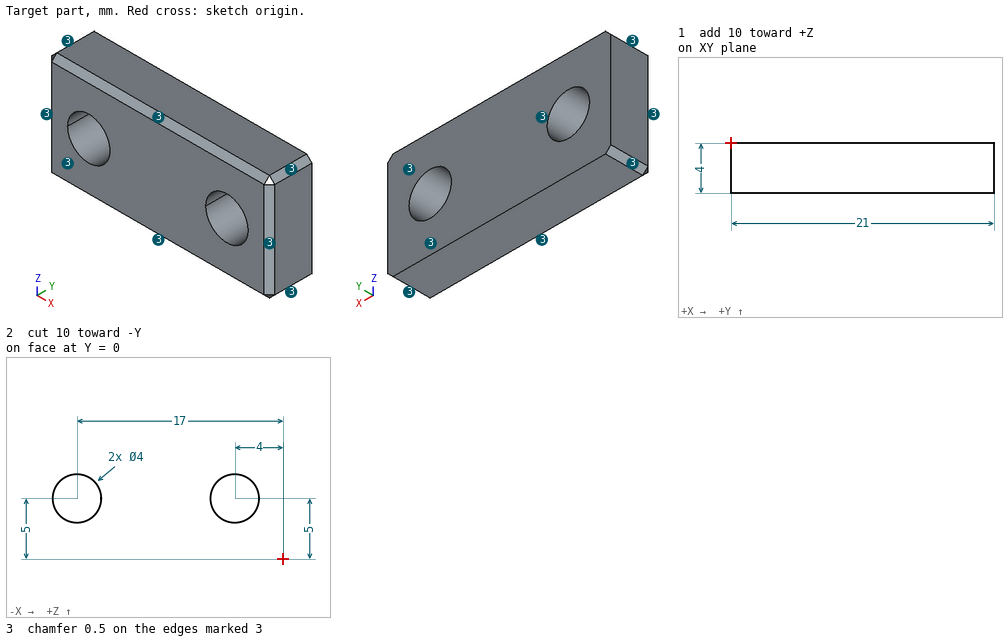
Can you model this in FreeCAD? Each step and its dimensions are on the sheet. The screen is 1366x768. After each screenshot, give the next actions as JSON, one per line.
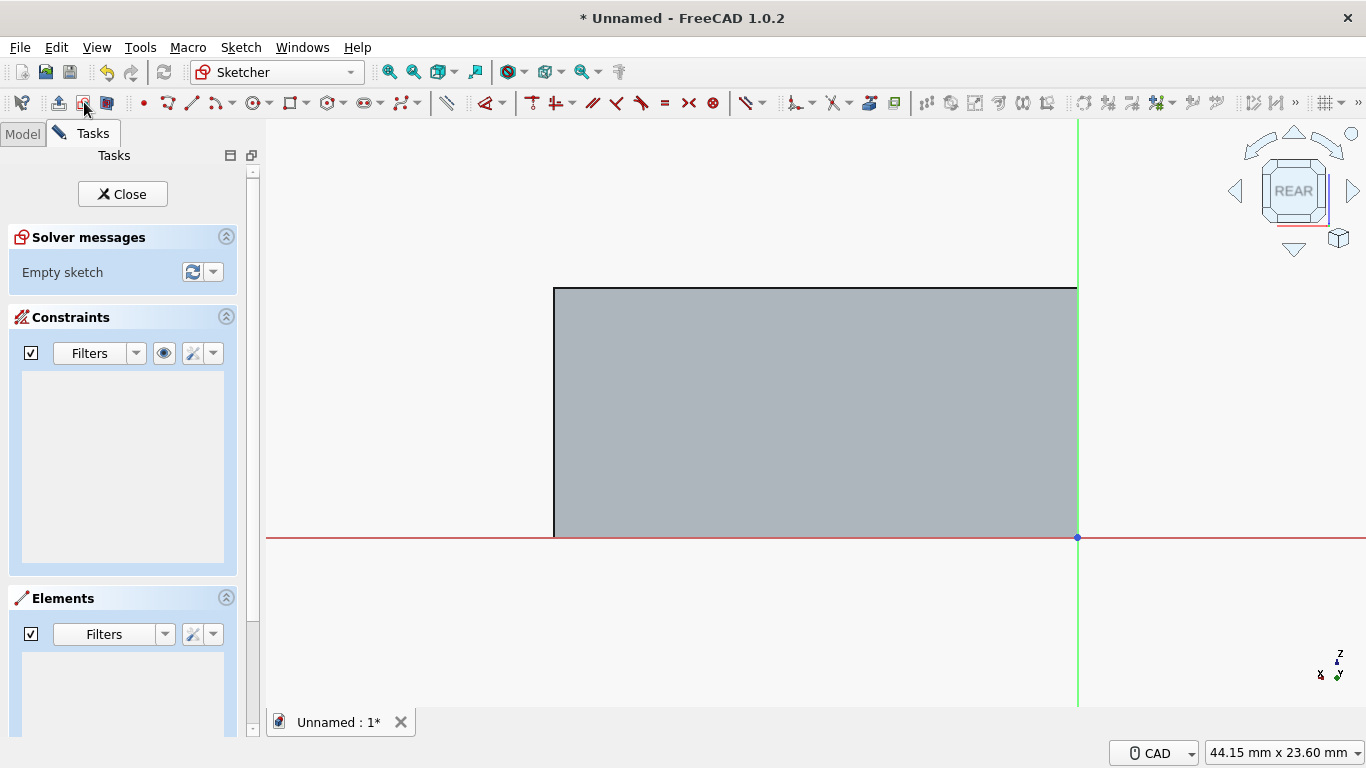
{"action": "scroll", "coordinate": [1031, 526], "scroll_direction": "up", "scroll_amount": 2}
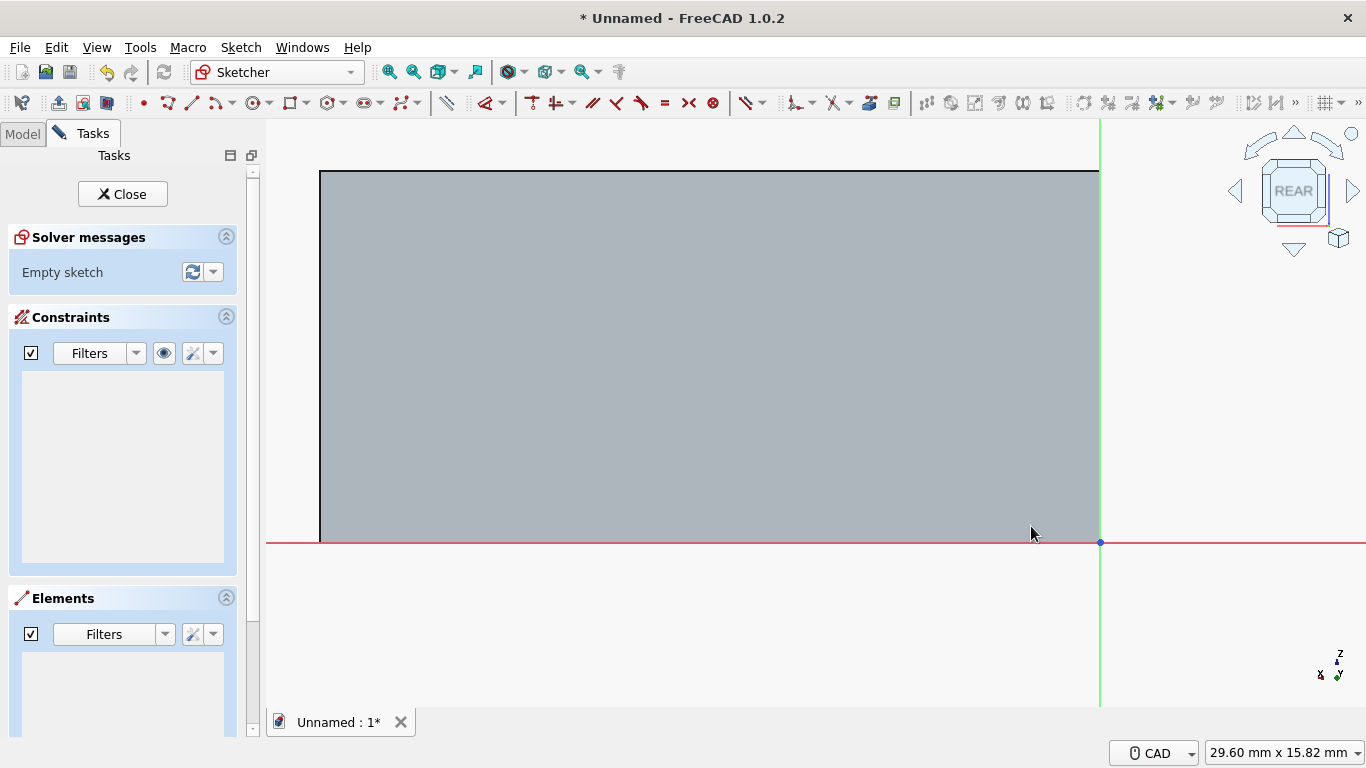
{"action": "left_click", "coordinate": [254, 104]}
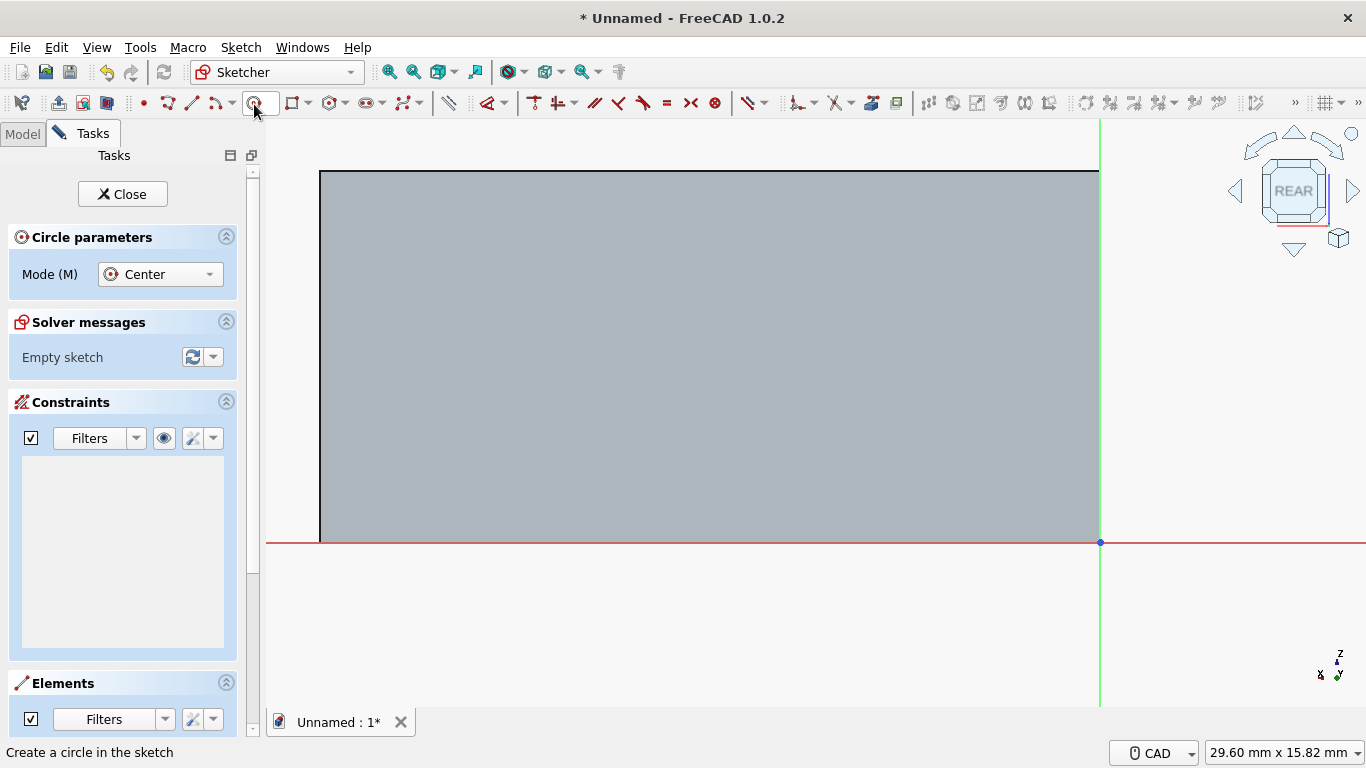
{"action": "left_click", "coordinate": [468, 357]}
{"action": "left_click", "coordinate": [521, 305]}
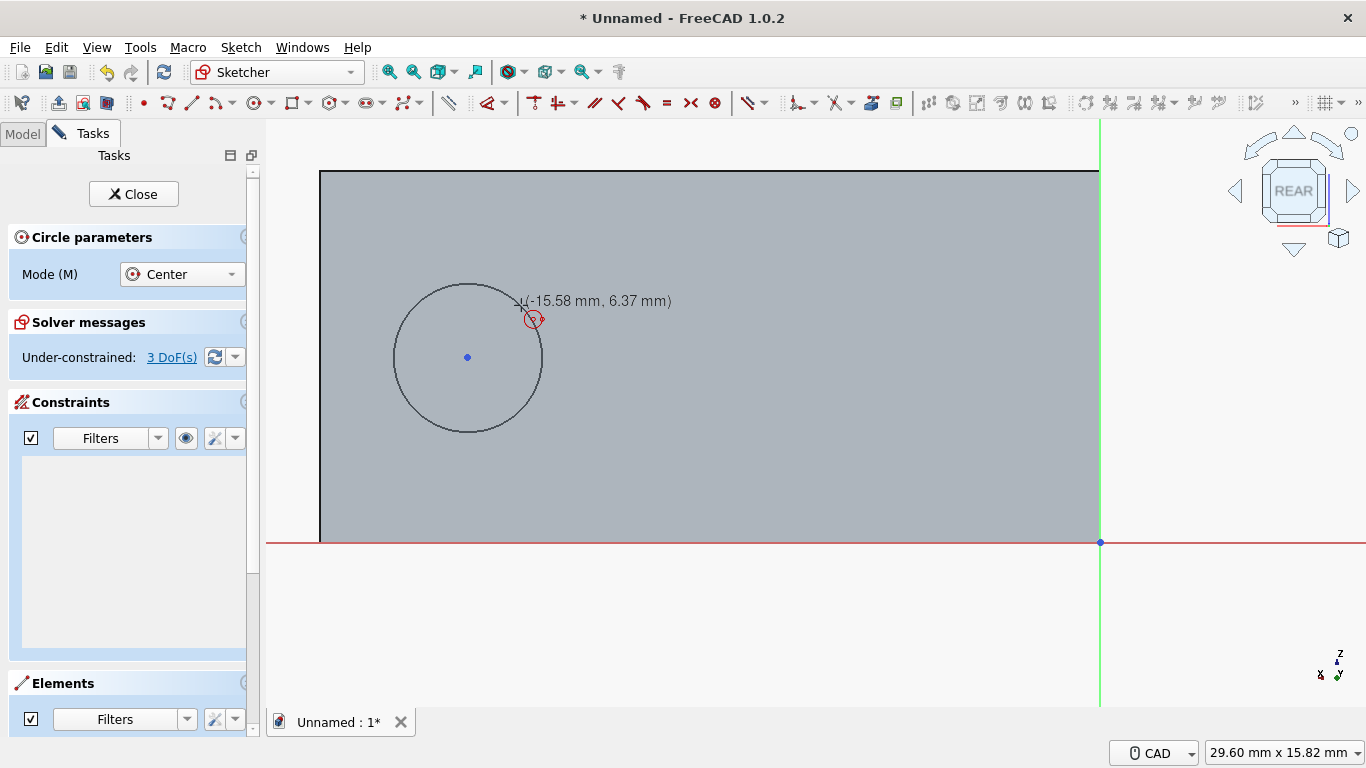
{"action": "left_click", "coordinate": [952, 357]}
{"action": "left_click", "coordinate": [1004, 305]}
{"action": "key", "text": "Escape"}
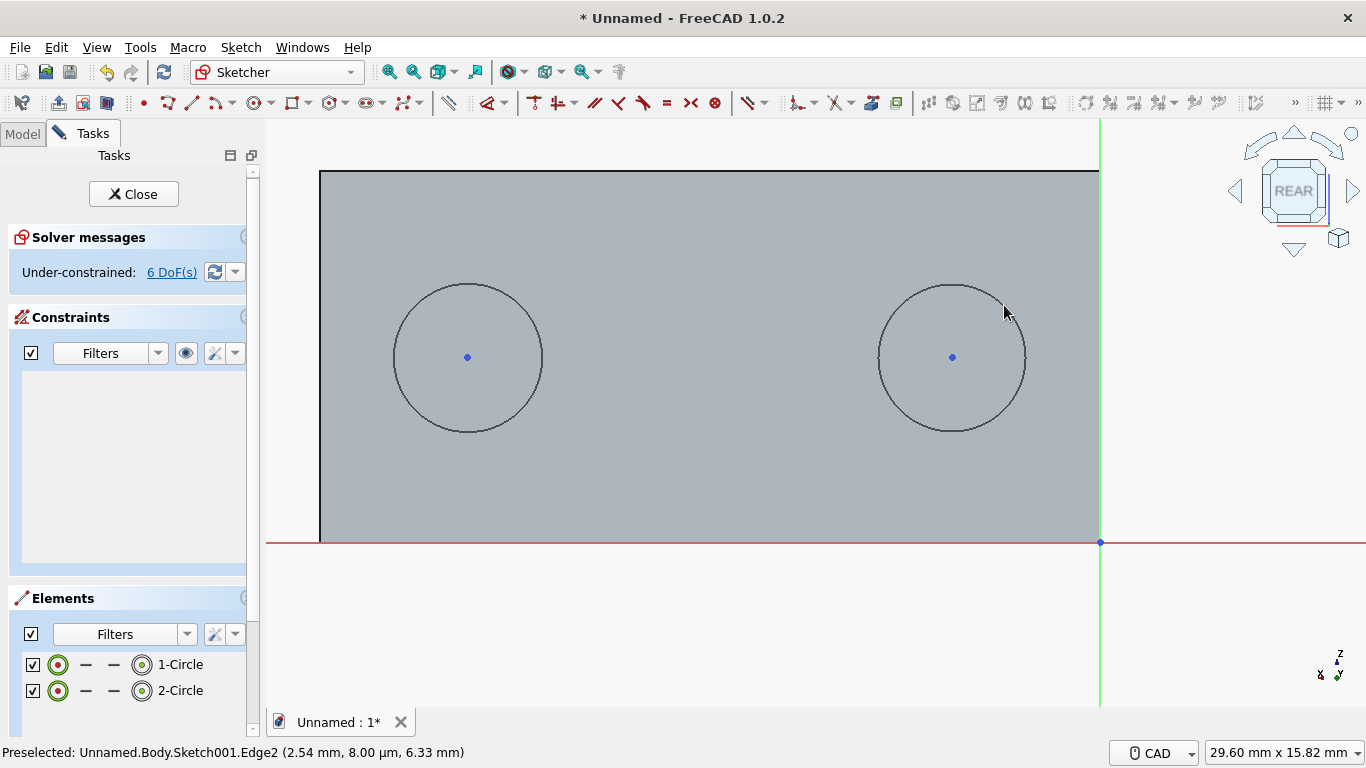
{"action": "left_click", "coordinate": [520, 305]}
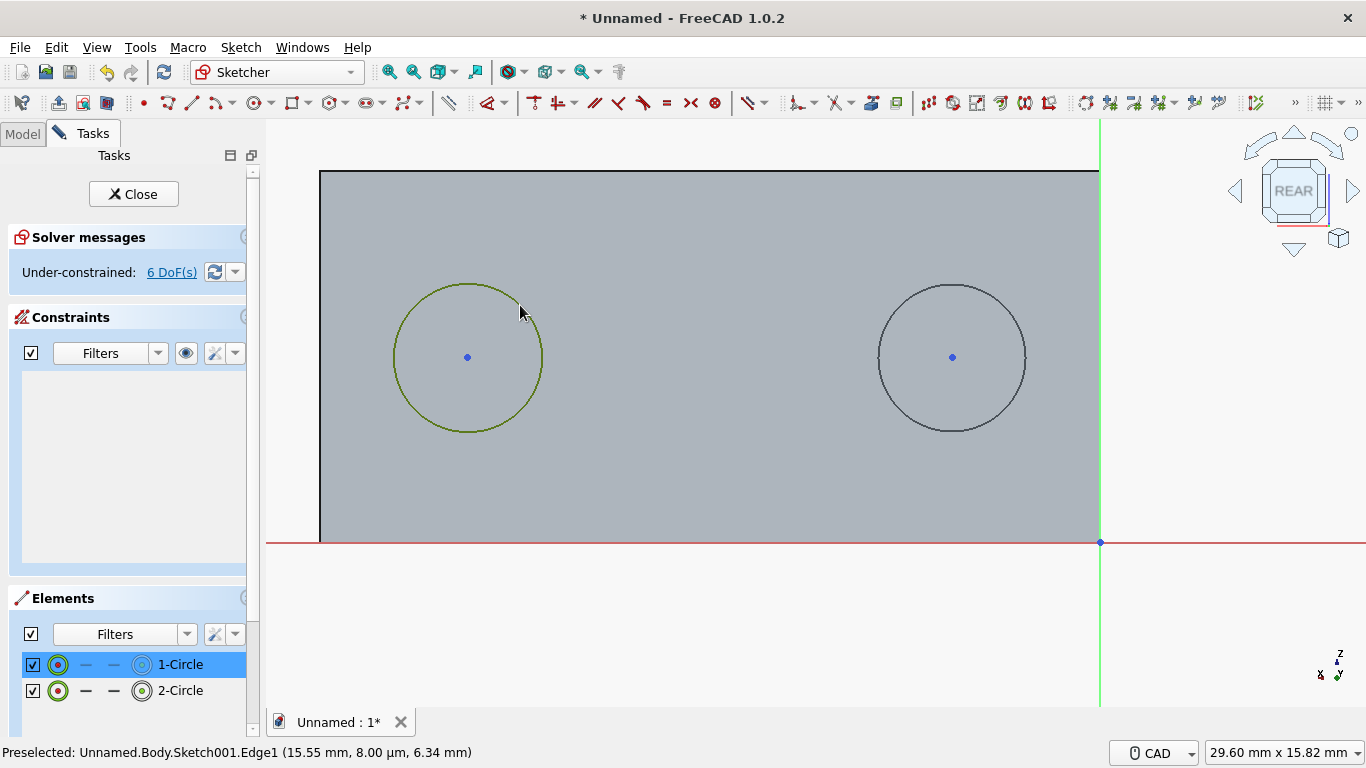
{"action": "left_click", "coordinate": [1004, 306]}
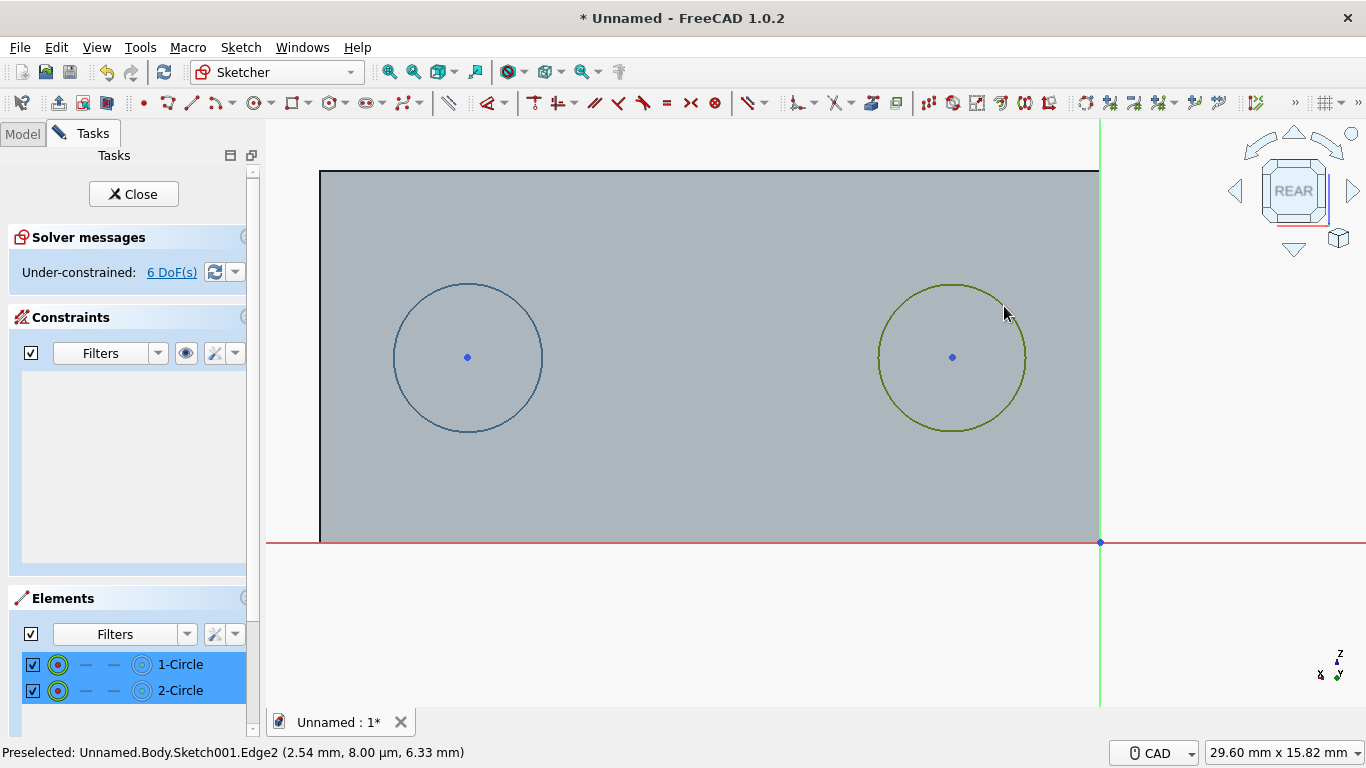
{"action": "left_click", "coordinate": [668, 104]}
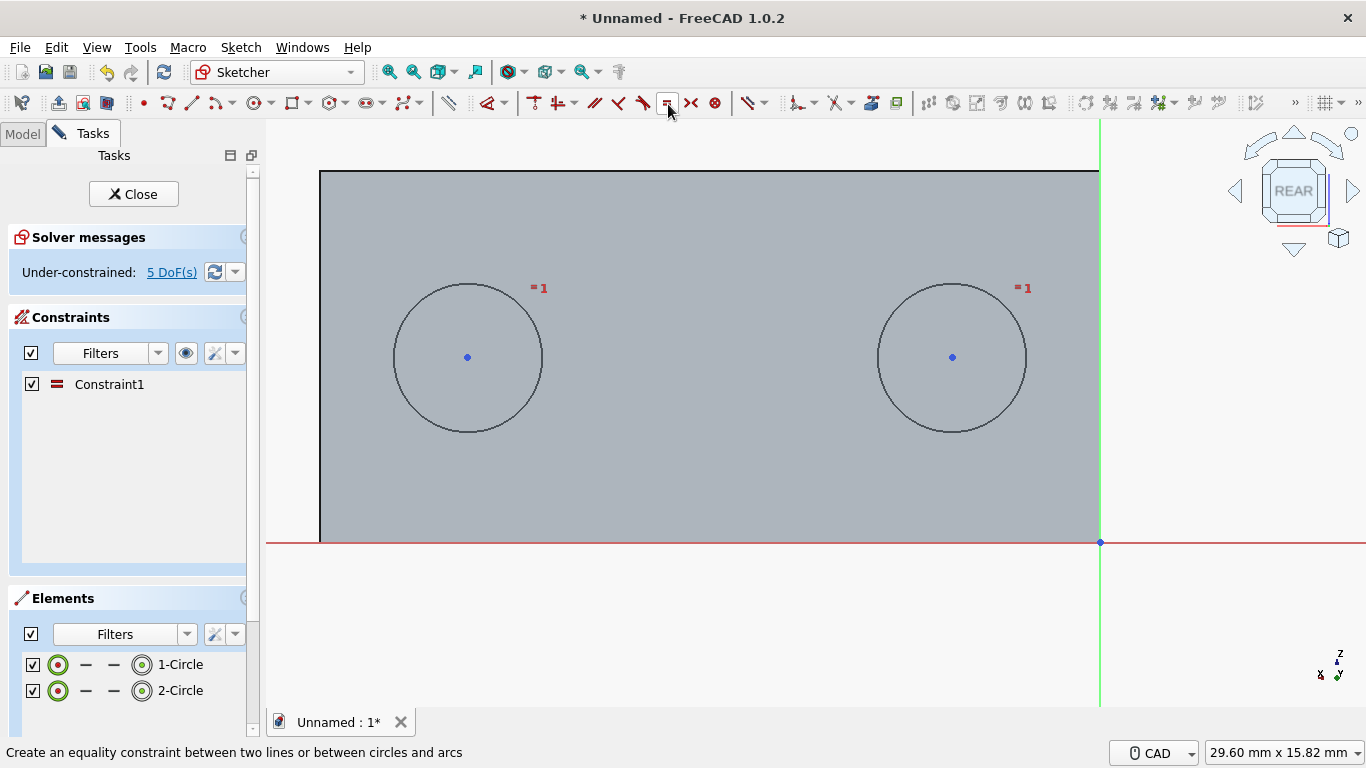
{"action": "left_click", "coordinate": [488, 104]}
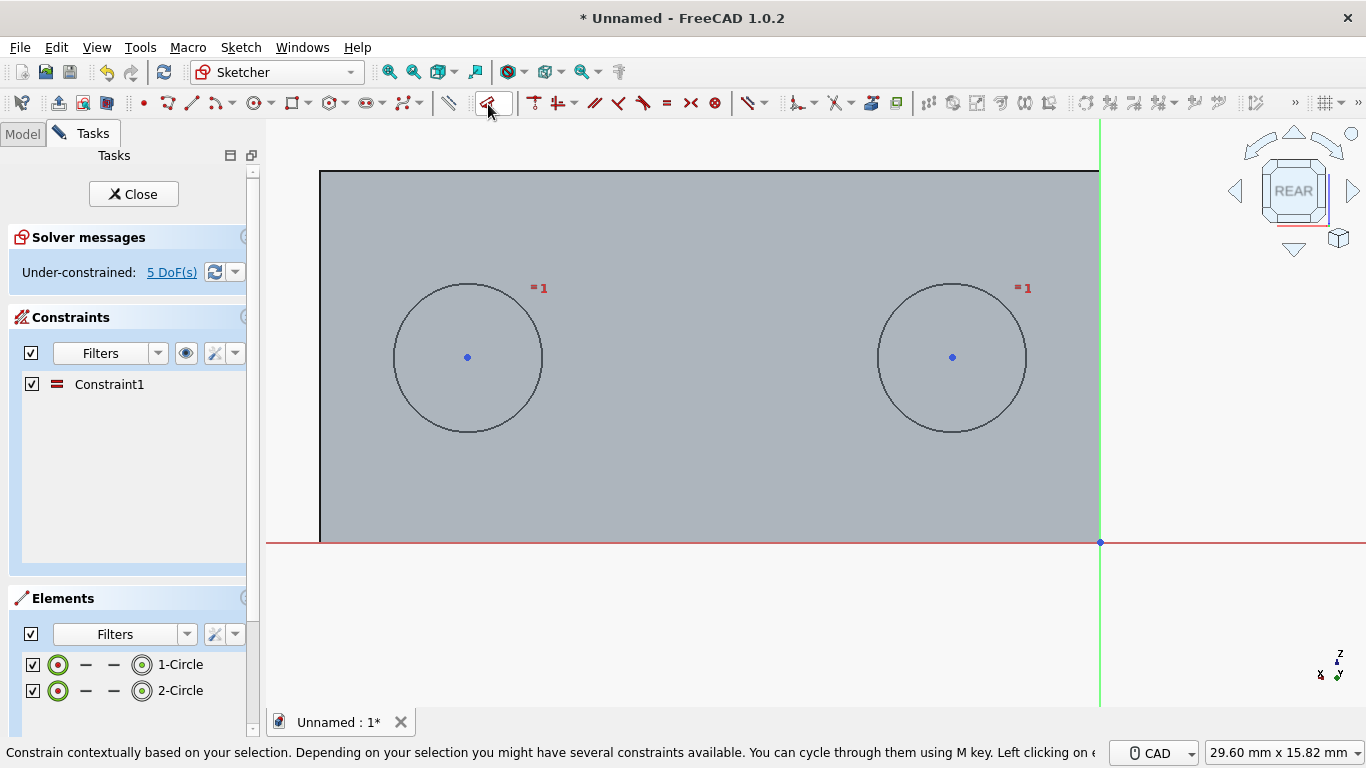
{"action": "left_click", "coordinate": [520, 305]}
{"action": "left_click", "coordinate": [542, 282]}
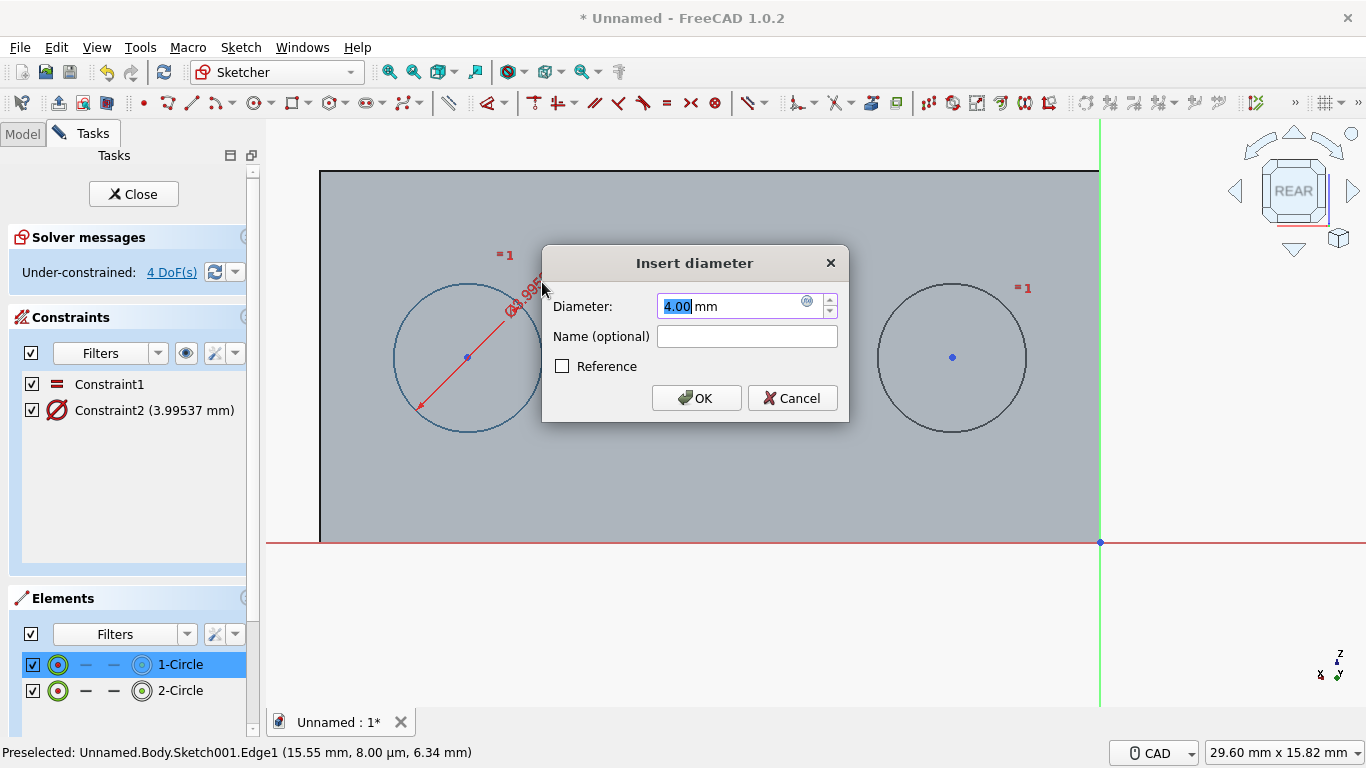
{"action": "type", "text": "4"}
{"action": "key", "text": "Return"}